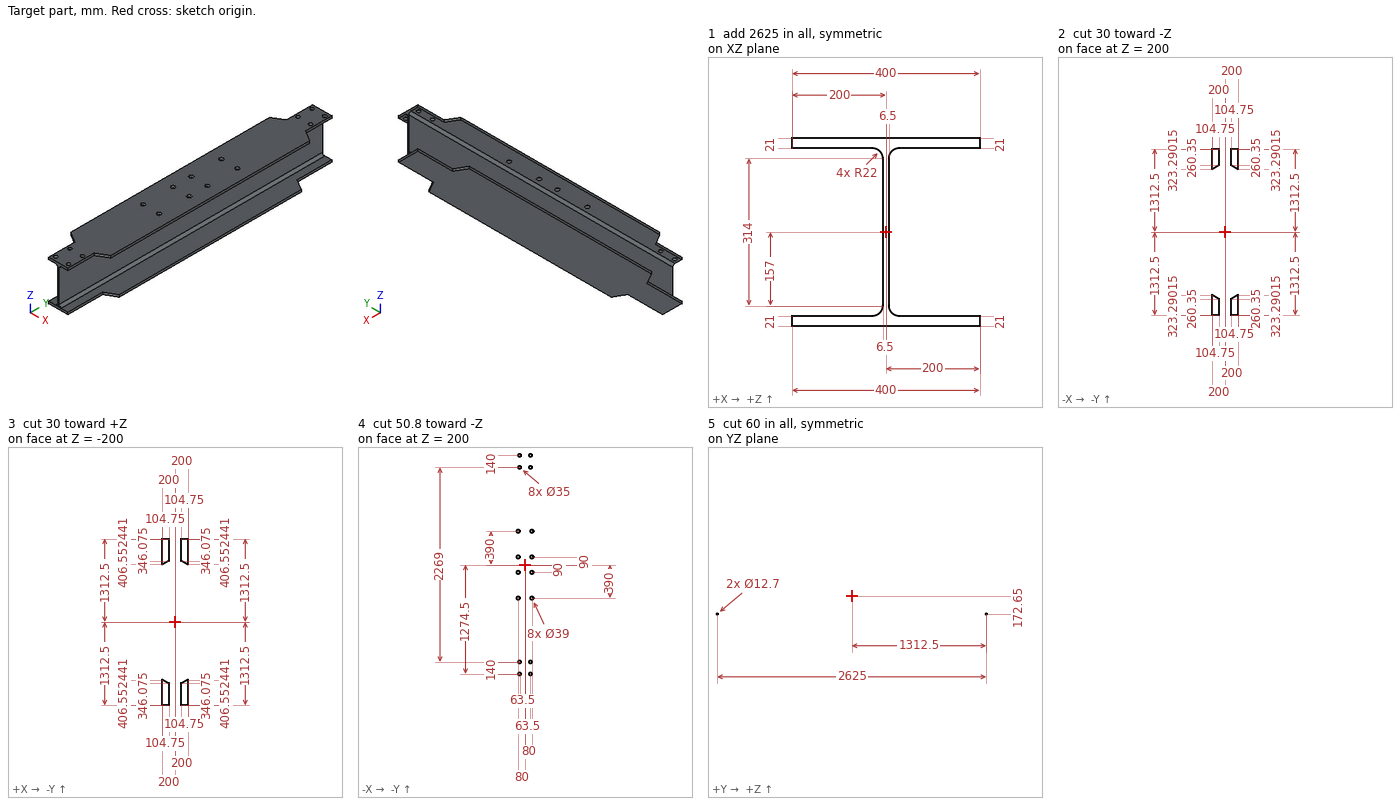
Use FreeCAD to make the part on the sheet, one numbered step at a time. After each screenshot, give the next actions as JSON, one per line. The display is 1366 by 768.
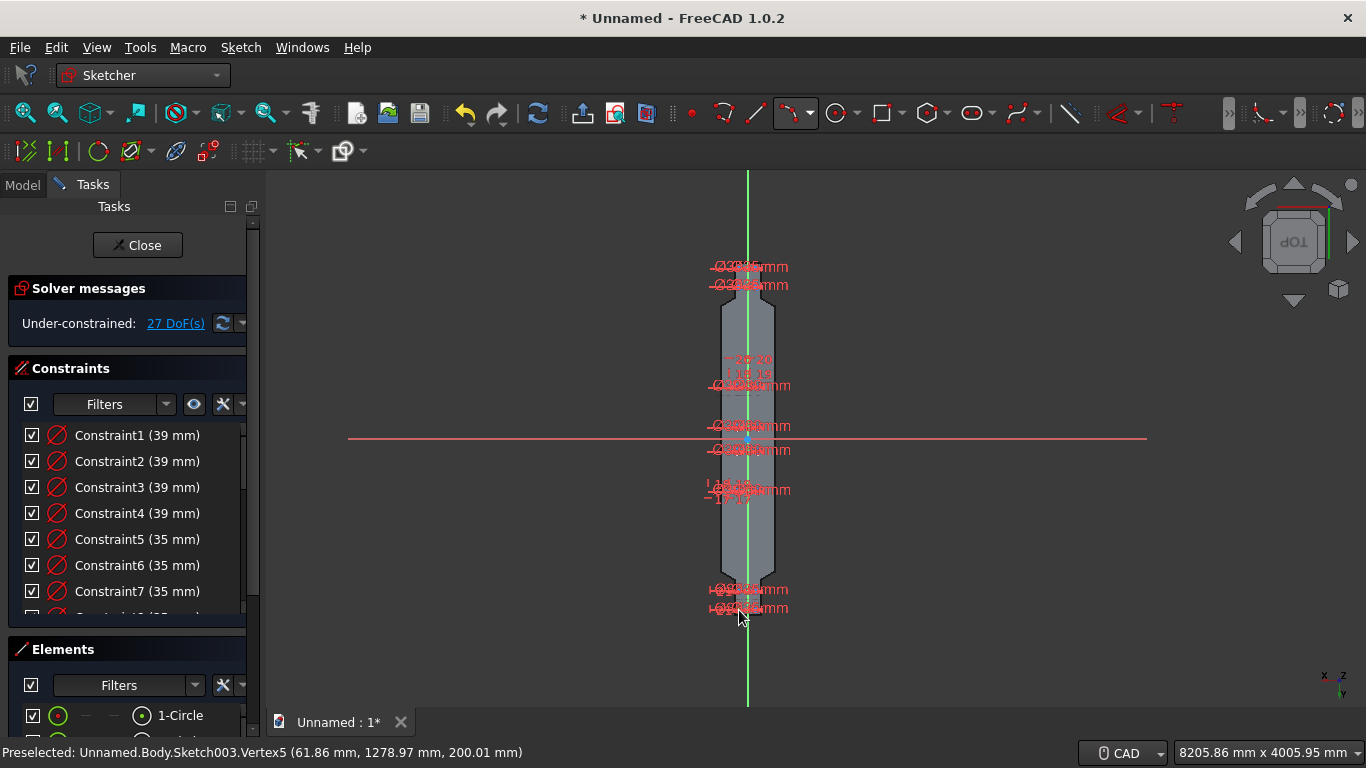
{"action": "left_click", "coordinate": [756, 610]}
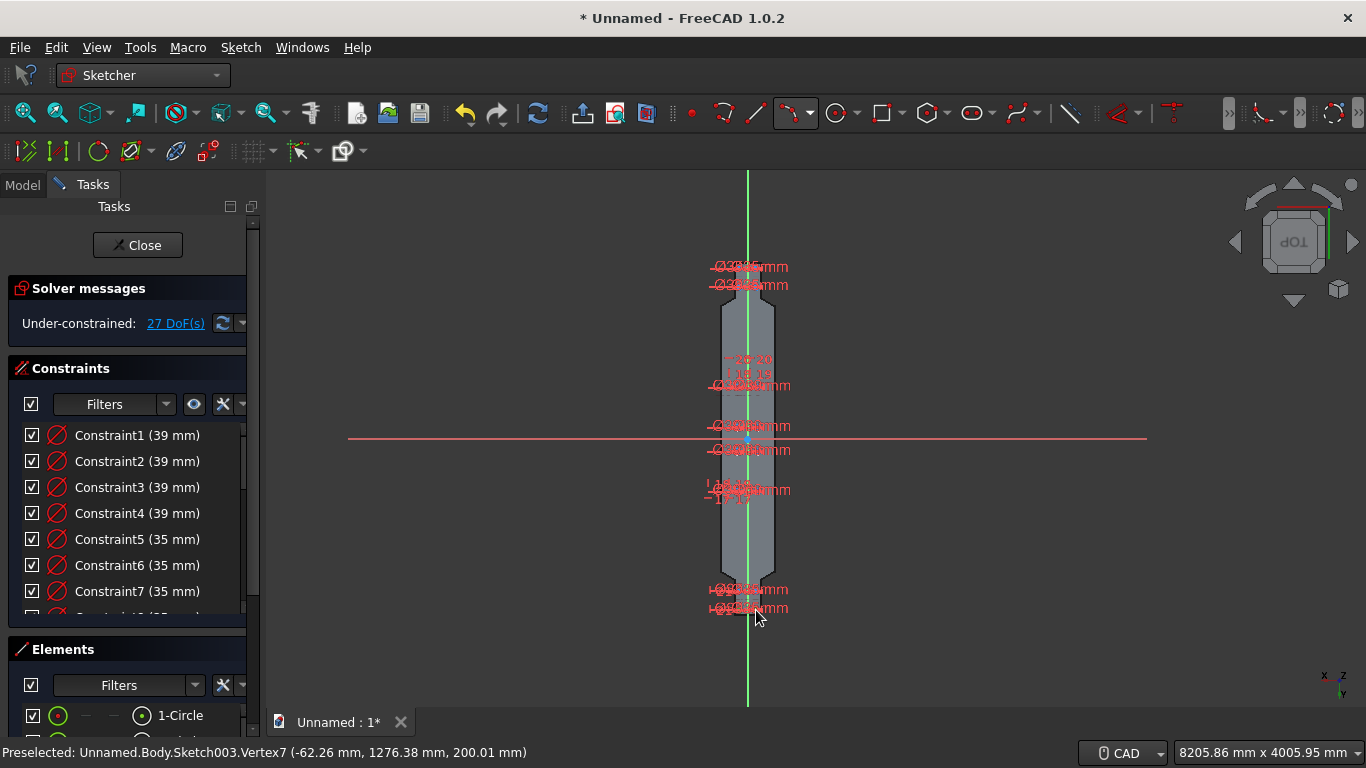
{"action": "key", "text": "h"}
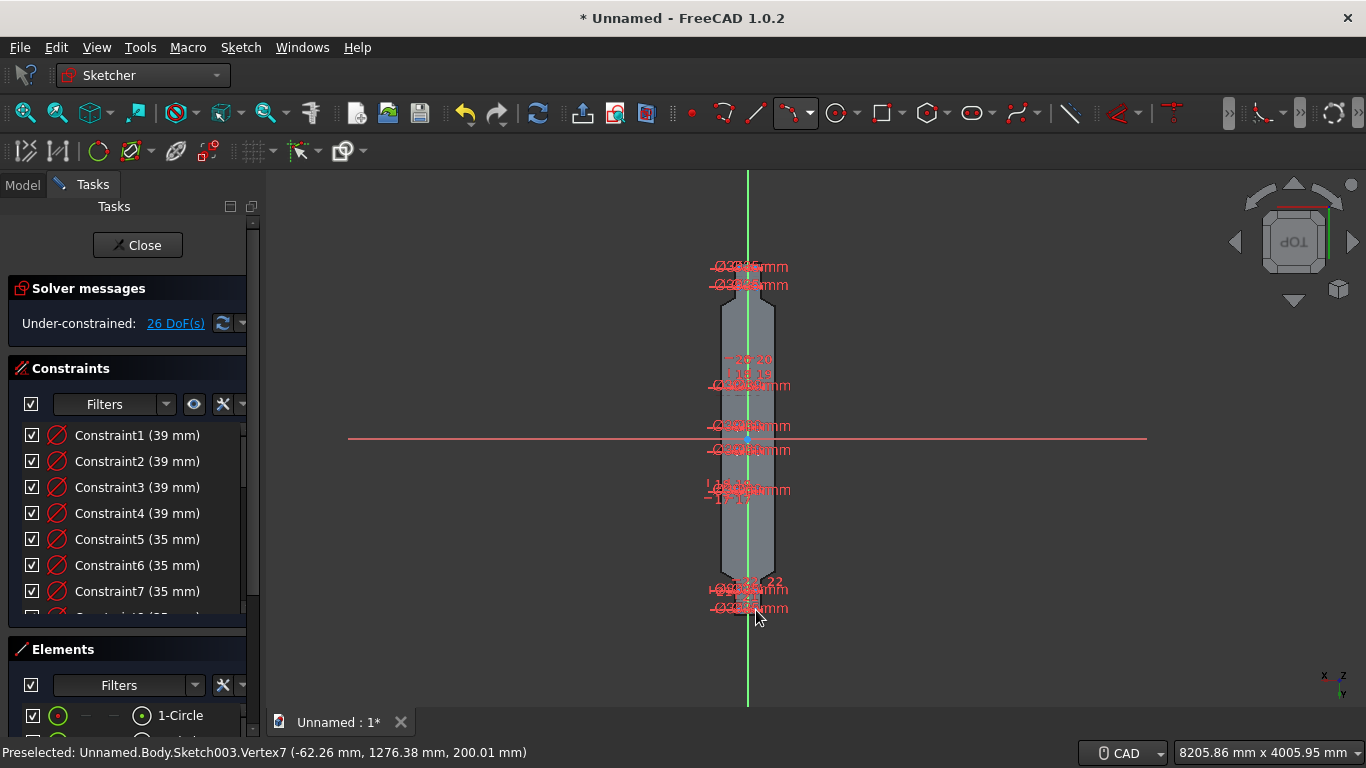
{"action": "left_click", "coordinate": [756, 610]}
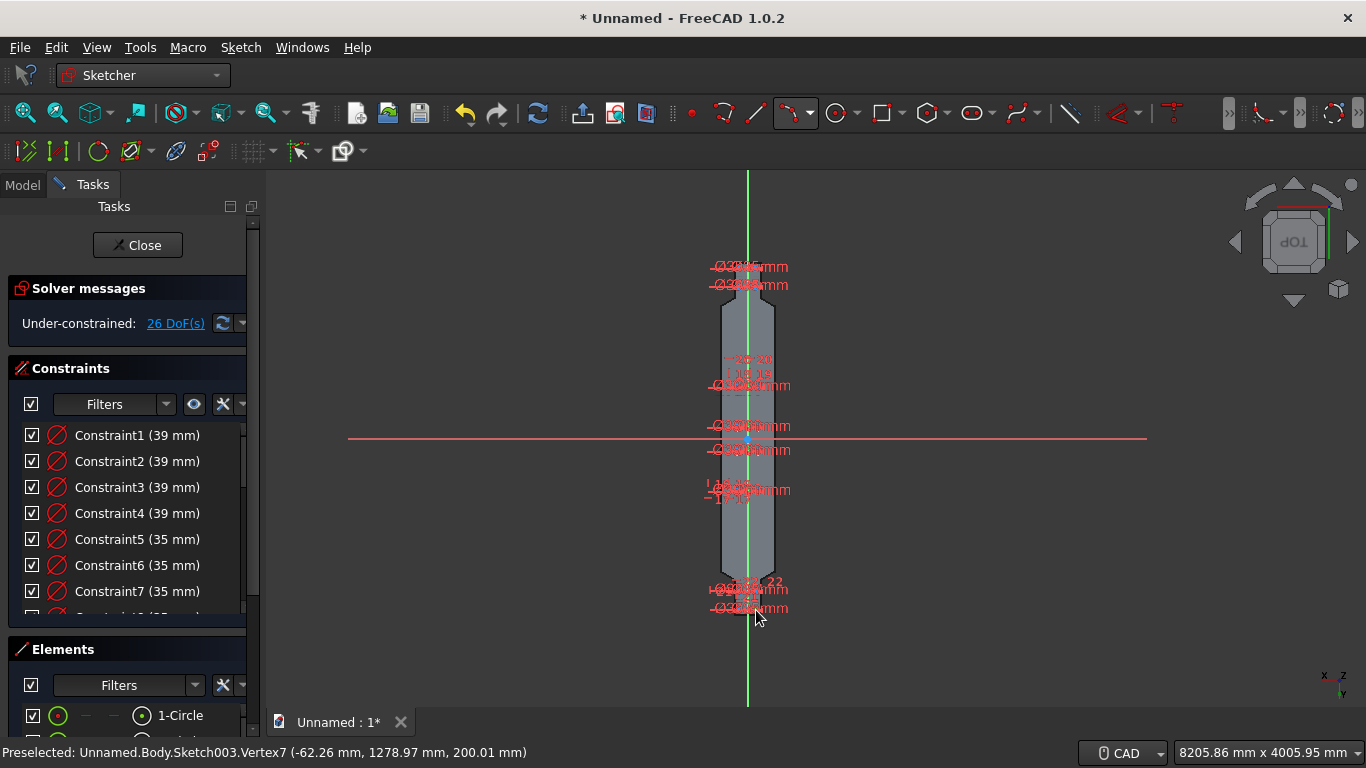
{"action": "scroll", "coordinate": [756, 592], "scroll_direction": "up", "scroll_amount": 4}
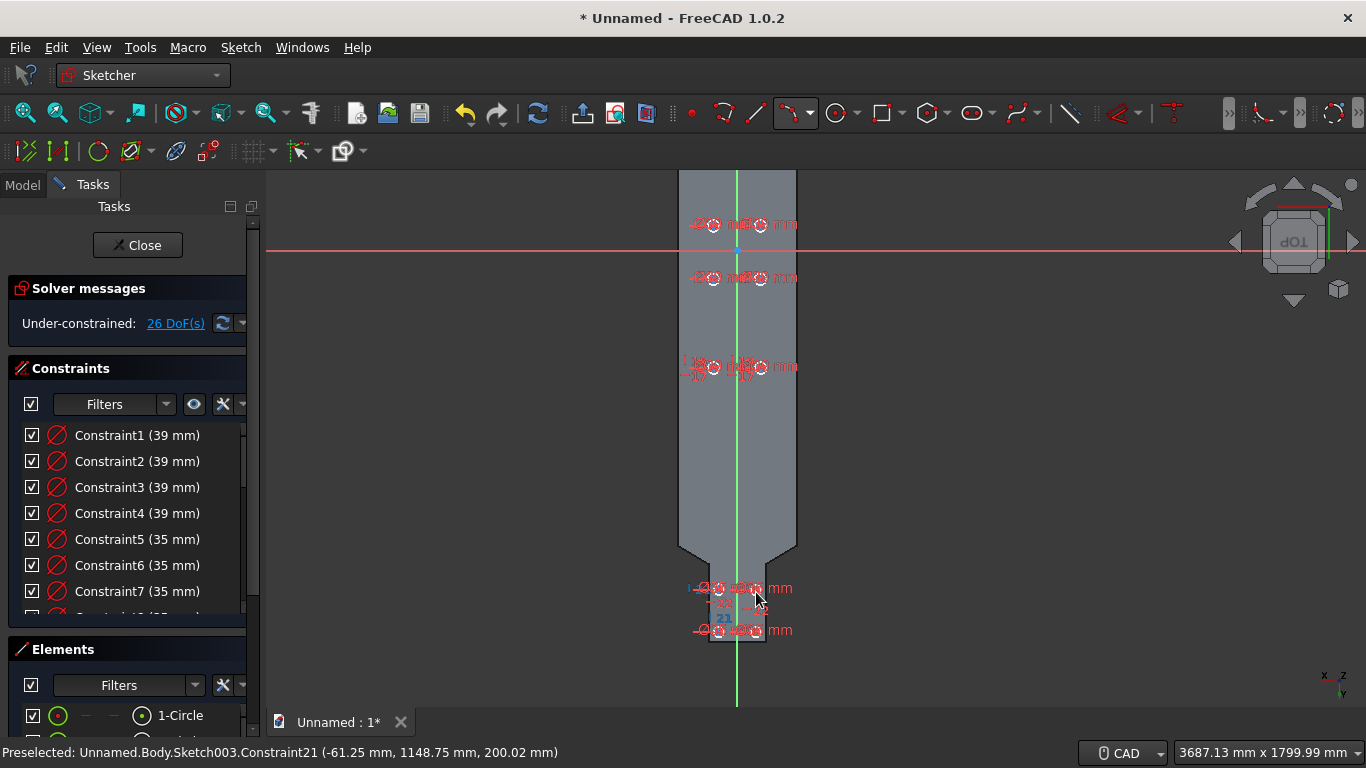
{"action": "left_click", "coordinate": [756, 590]}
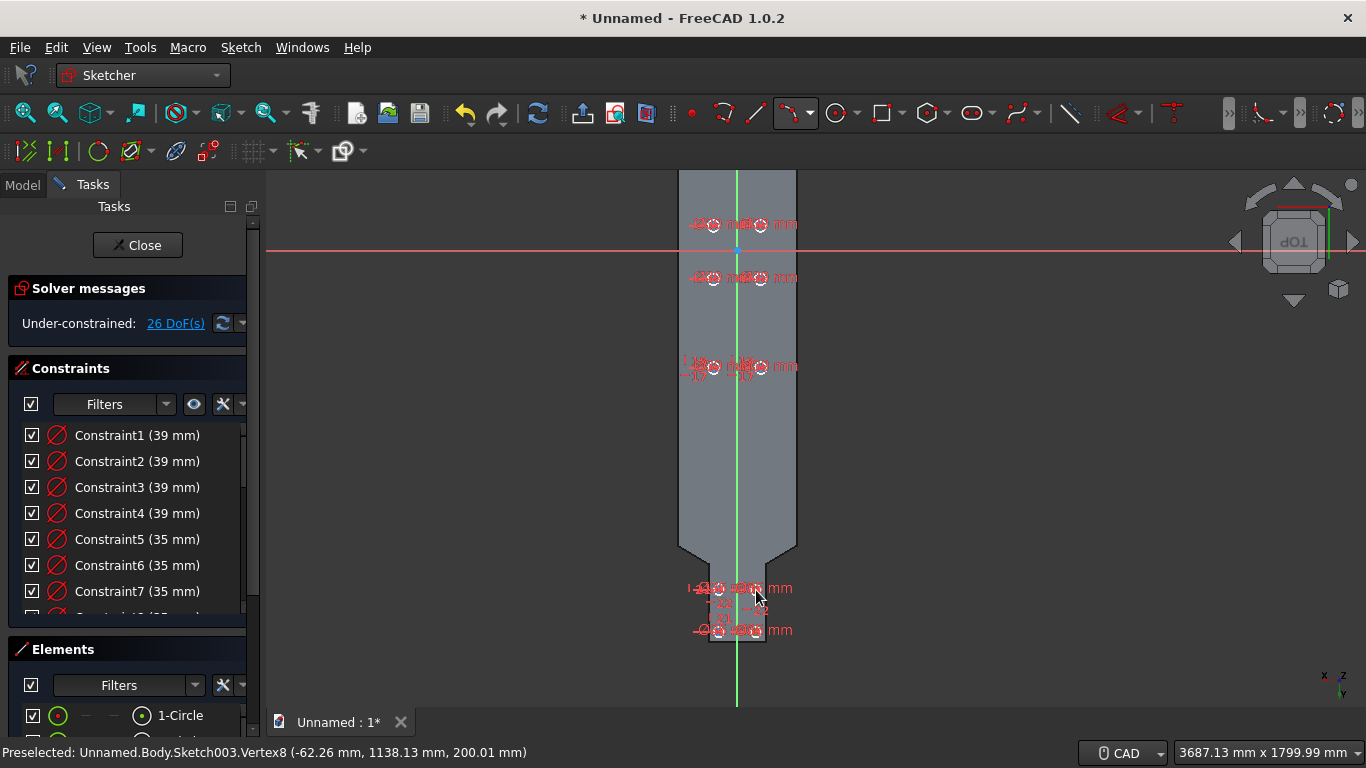
{"action": "key", "text": "v"}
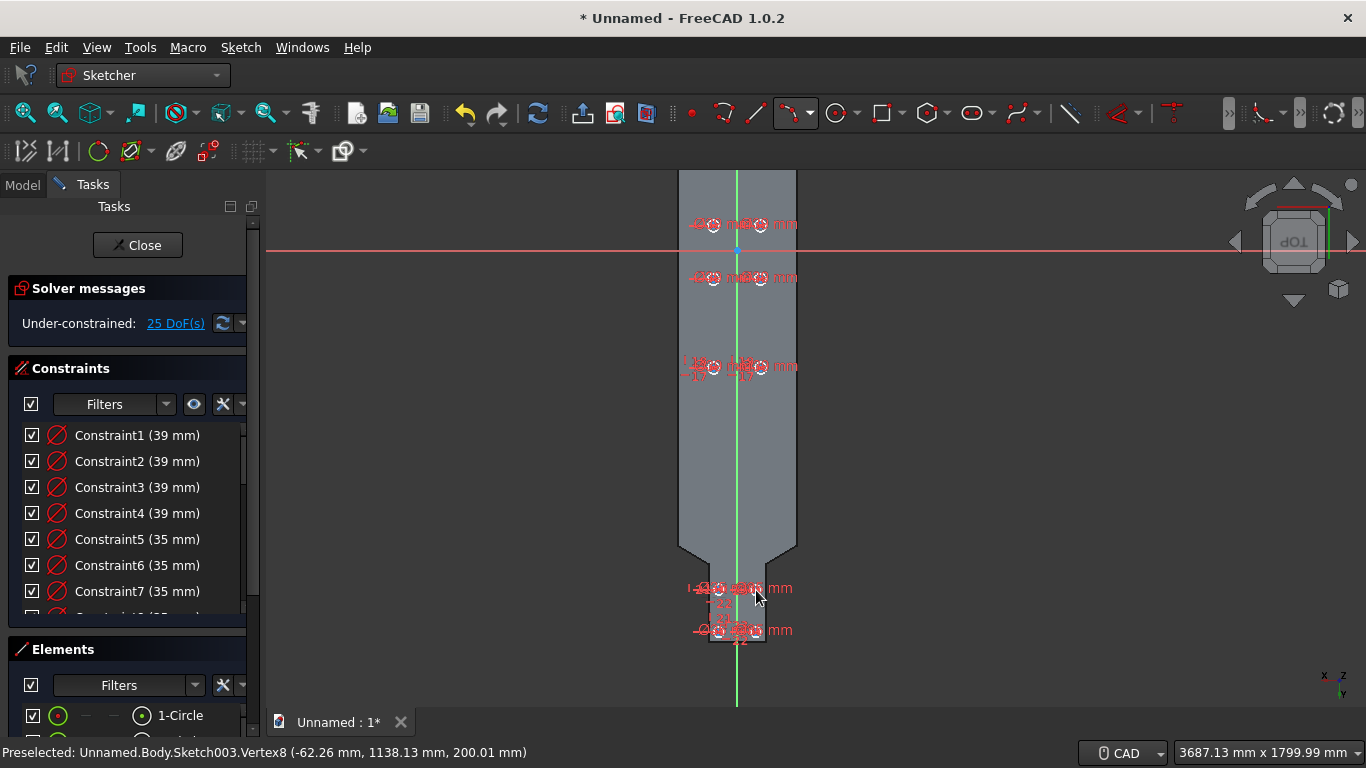
{"action": "left_click", "coordinate": [719, 590]}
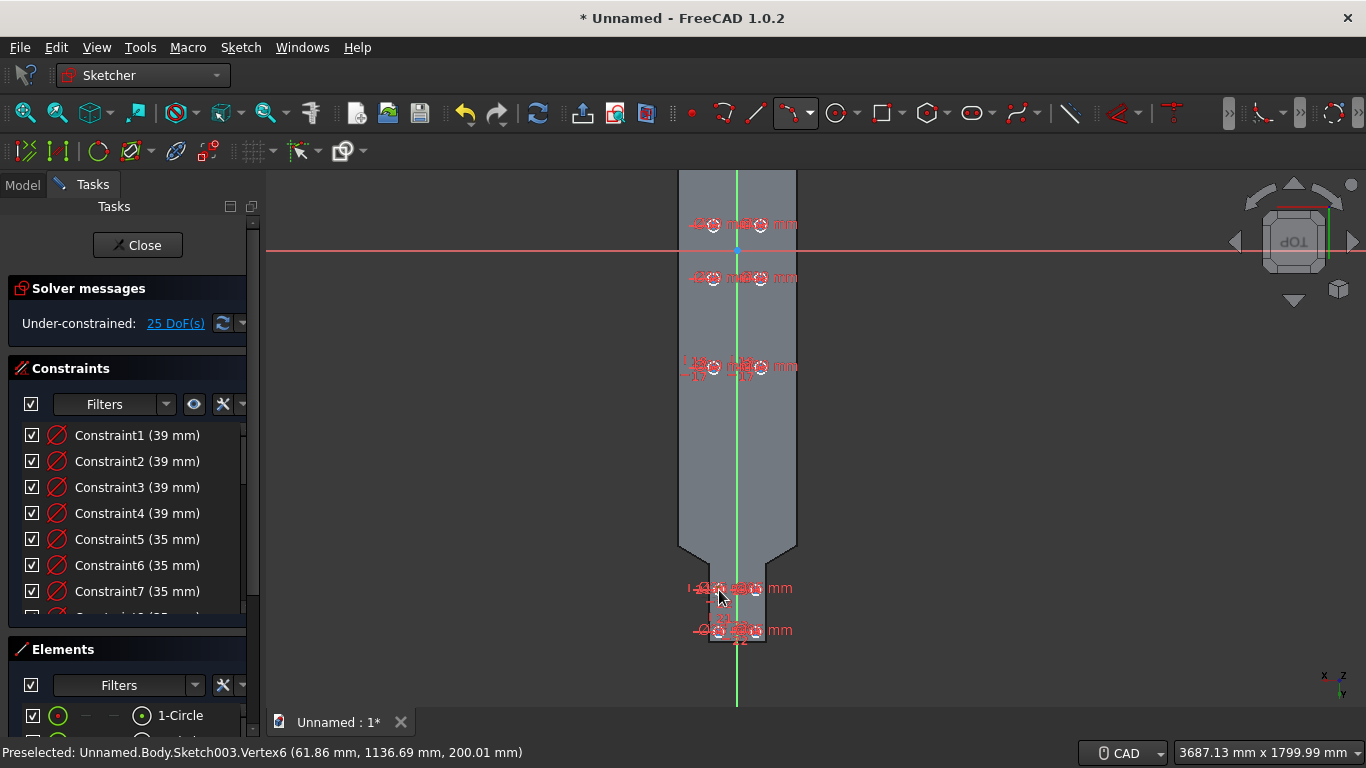
{"action": "left_click", "coordinate": [756, 590]}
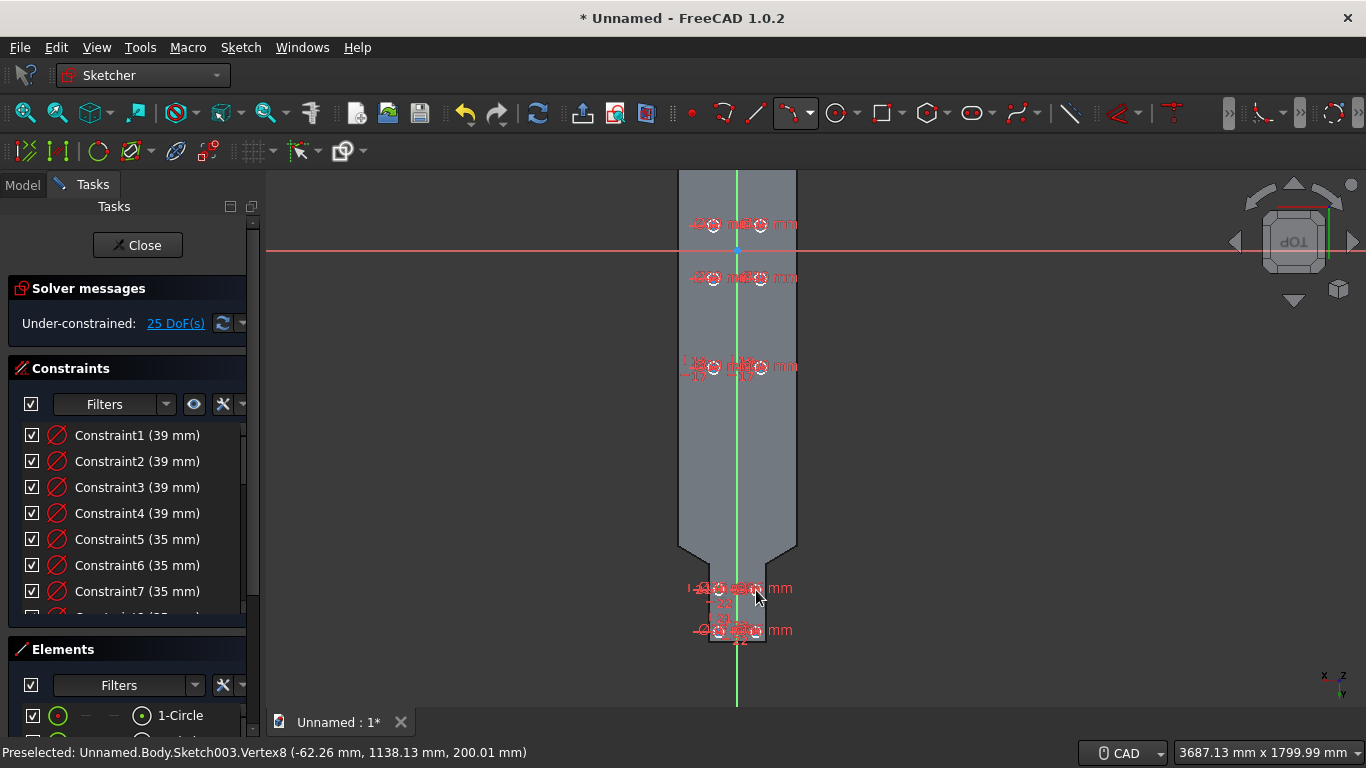
{"action": "key", "text": "h"}